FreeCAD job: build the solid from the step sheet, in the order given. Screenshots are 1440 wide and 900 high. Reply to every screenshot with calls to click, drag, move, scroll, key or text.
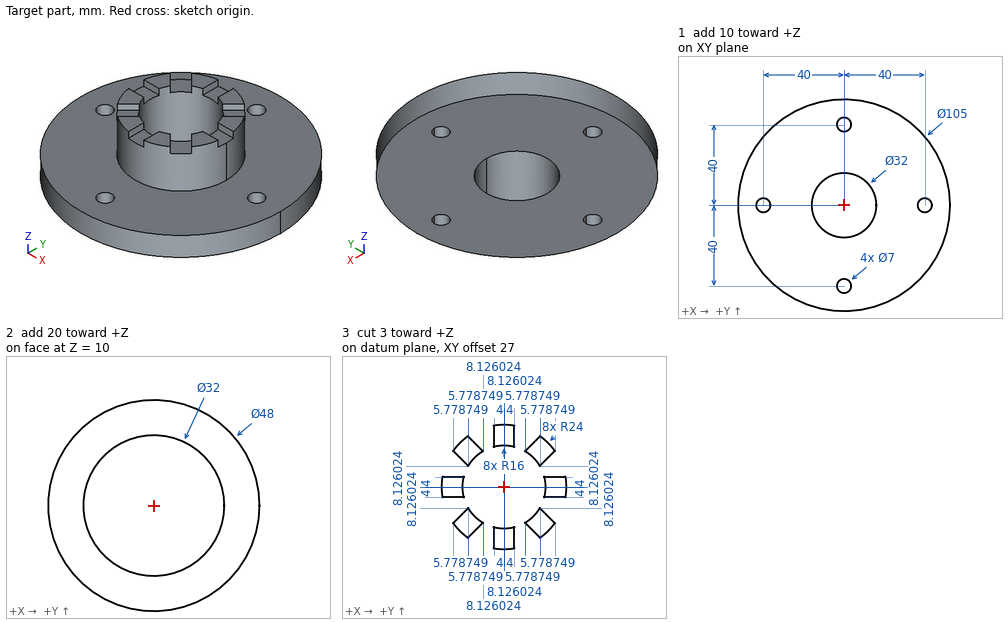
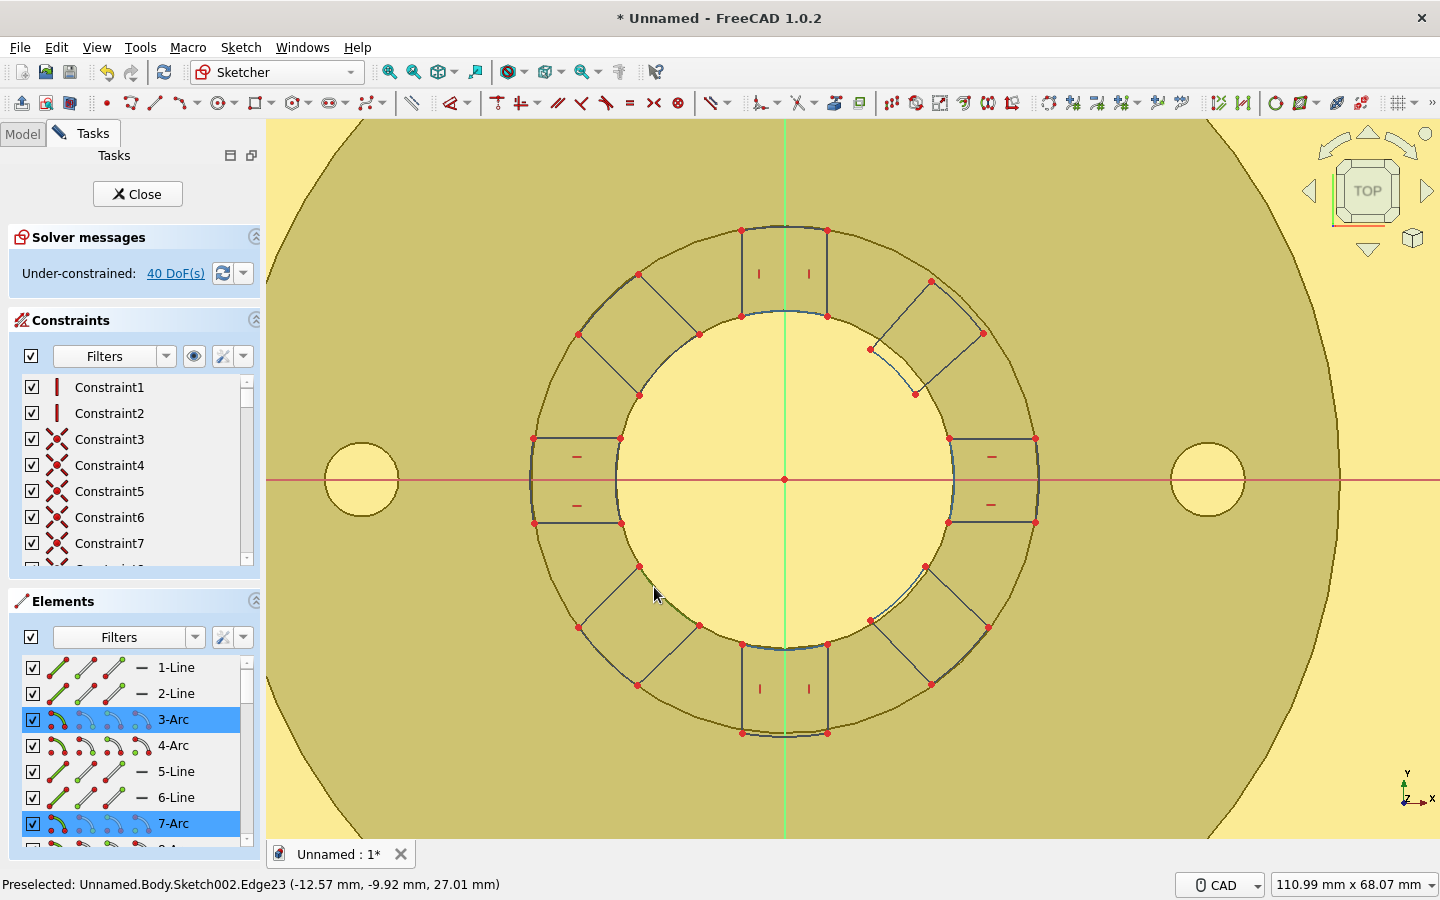
click(616, 464)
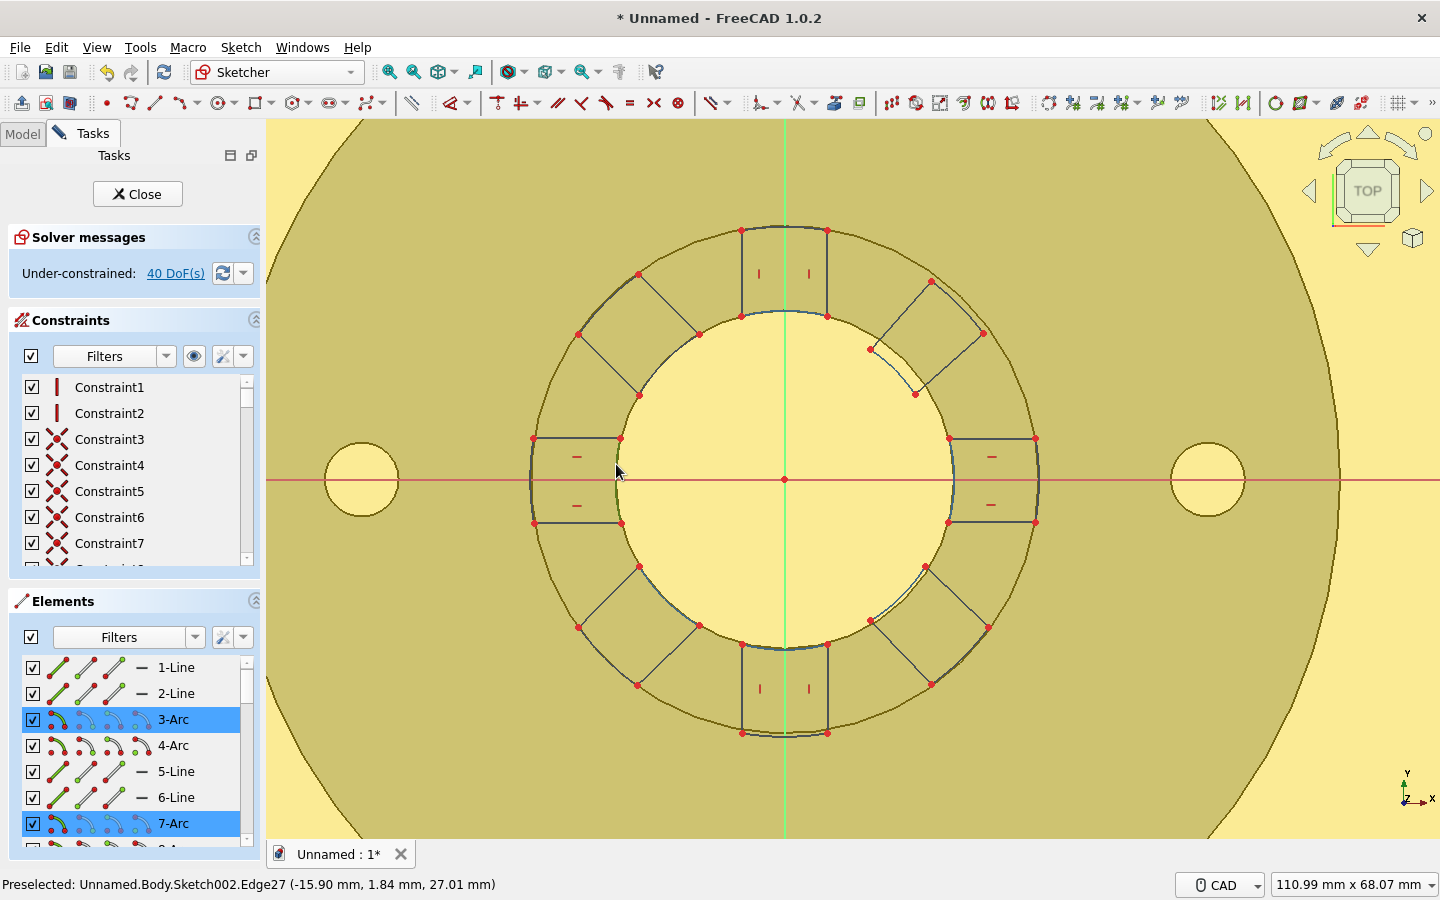
click(678, 349)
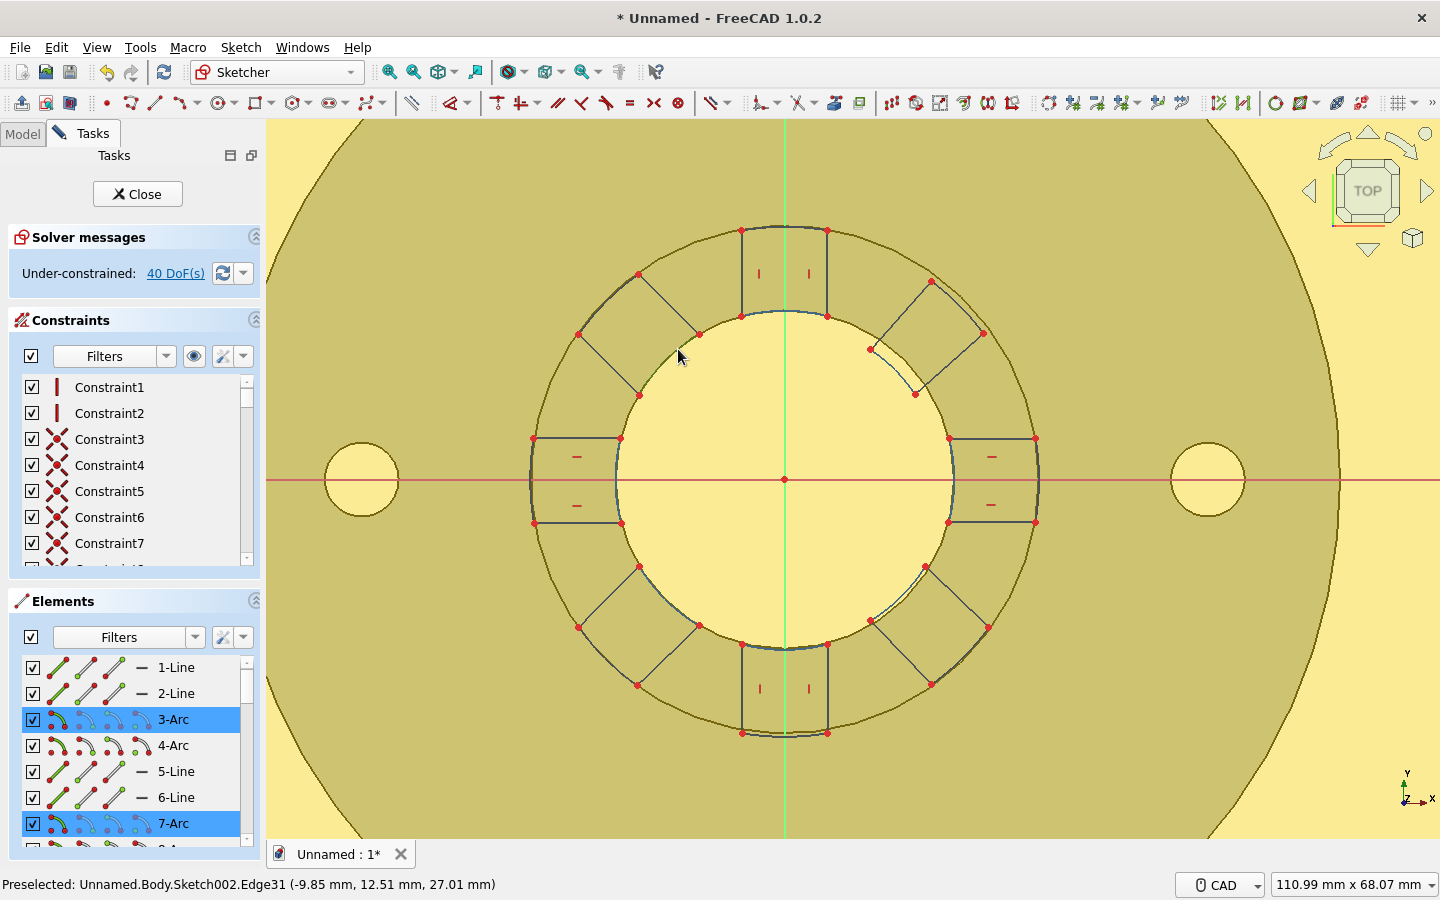
click(630, 104)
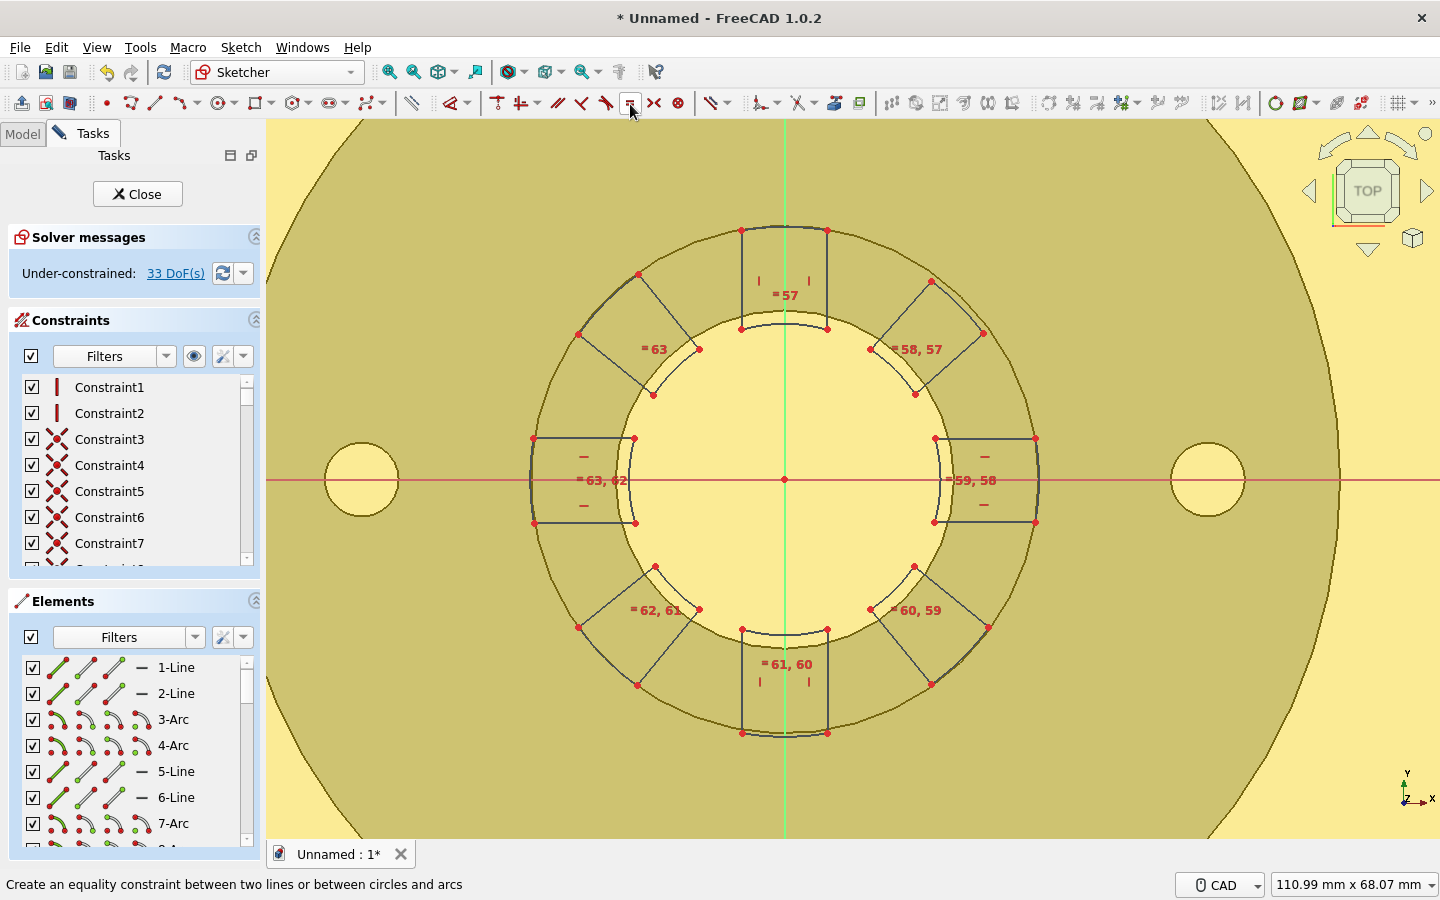
click(802, 227)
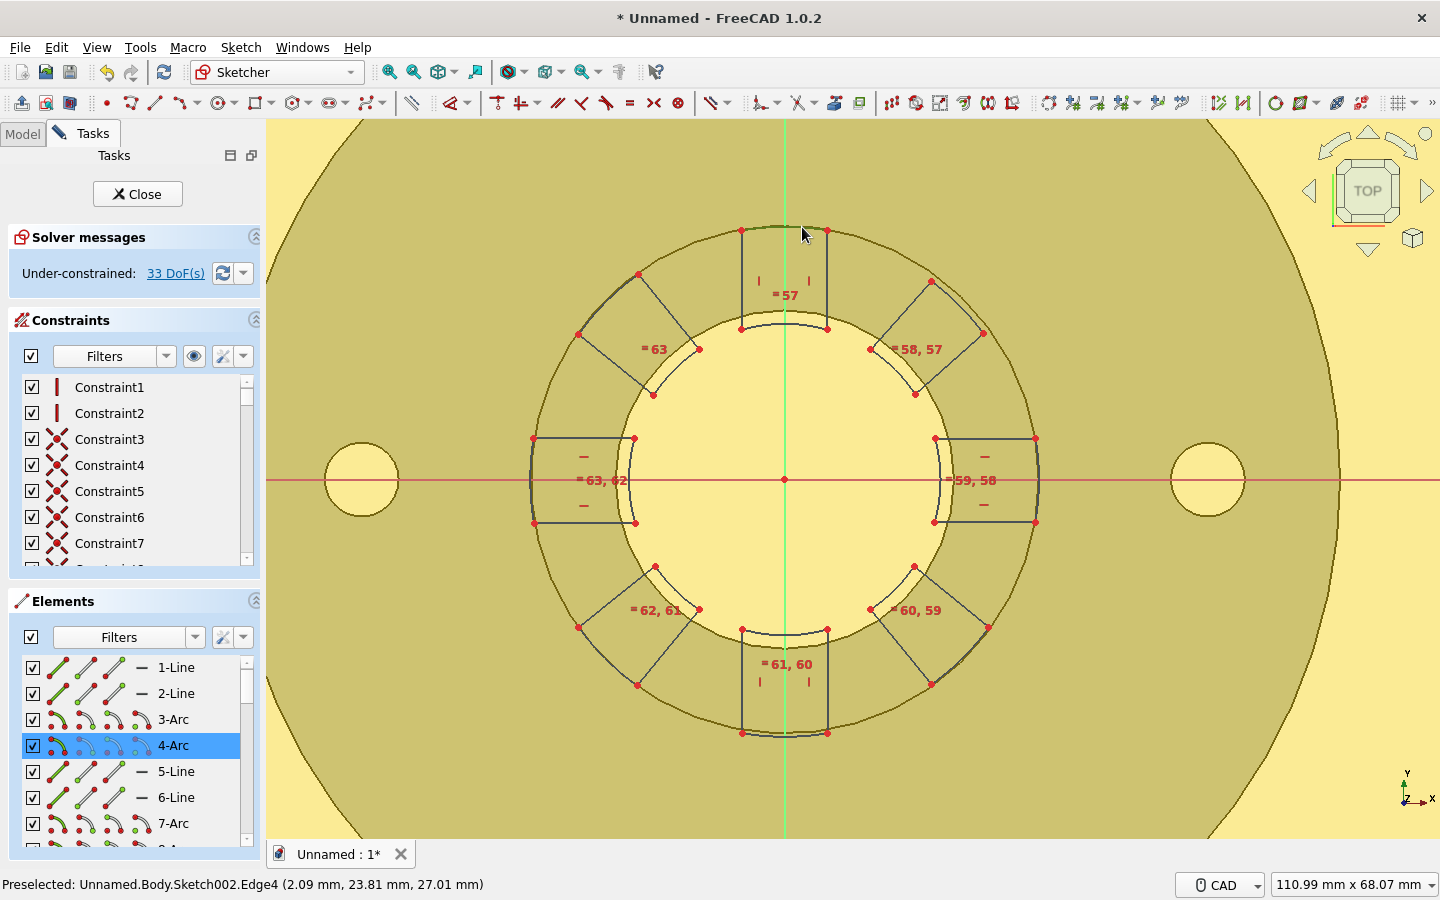
click(970, 316)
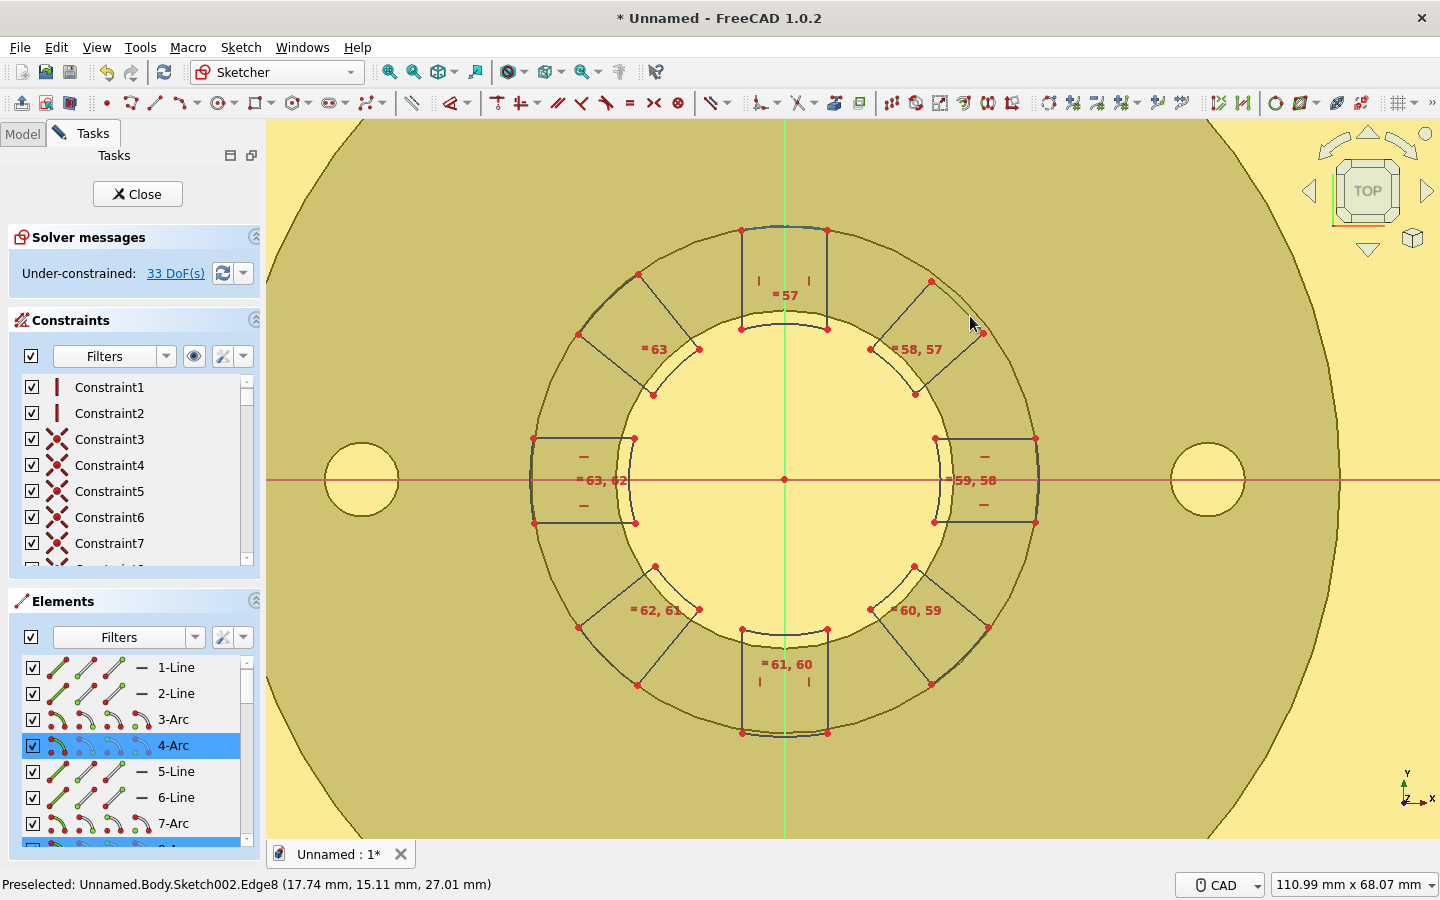
click(1038, 497)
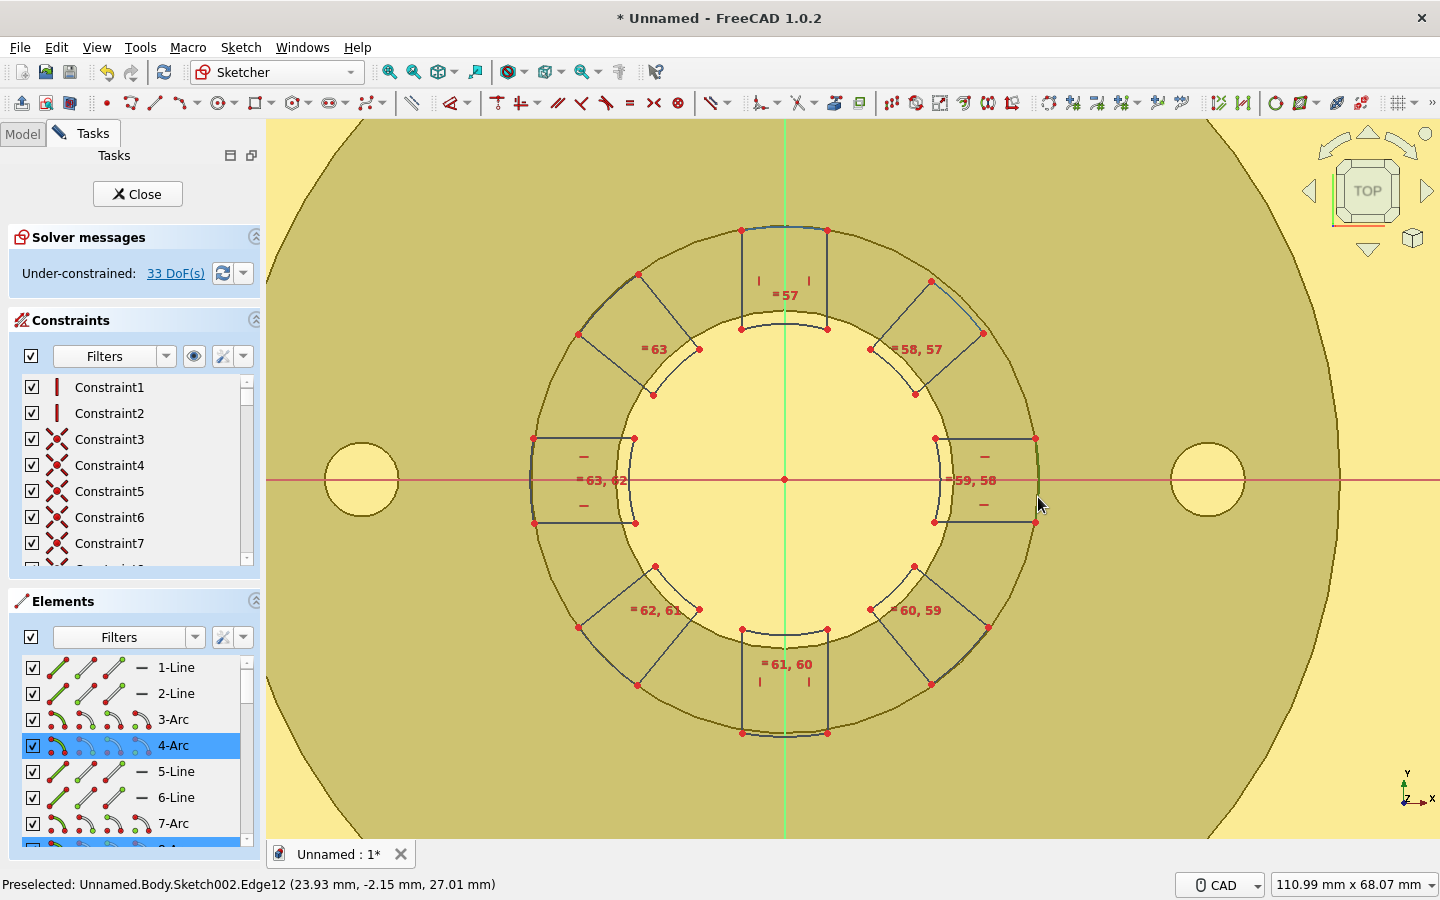
click(951, 669)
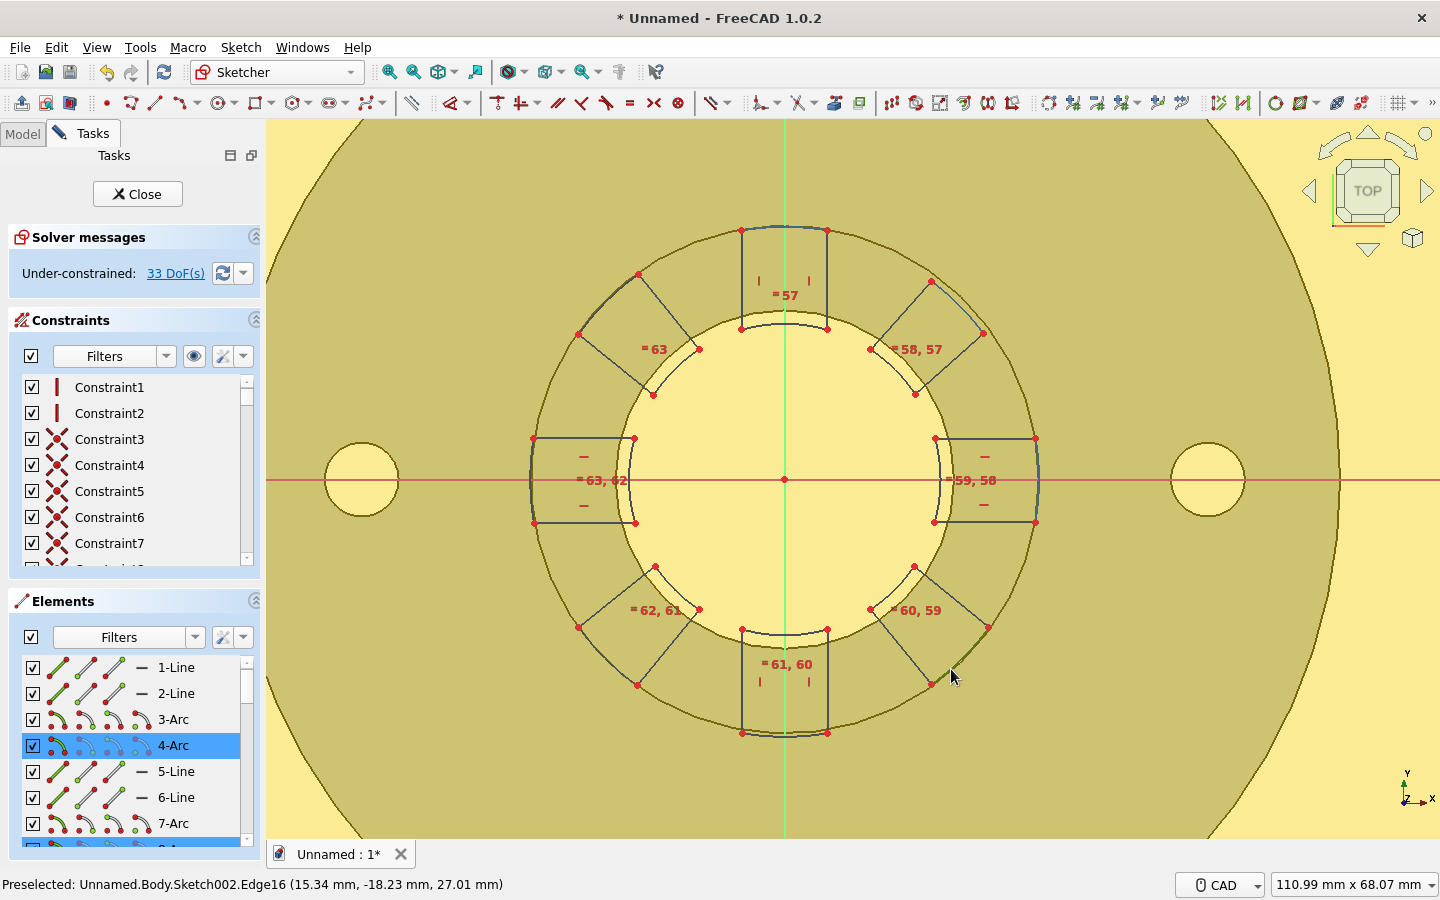
click(768, 736)